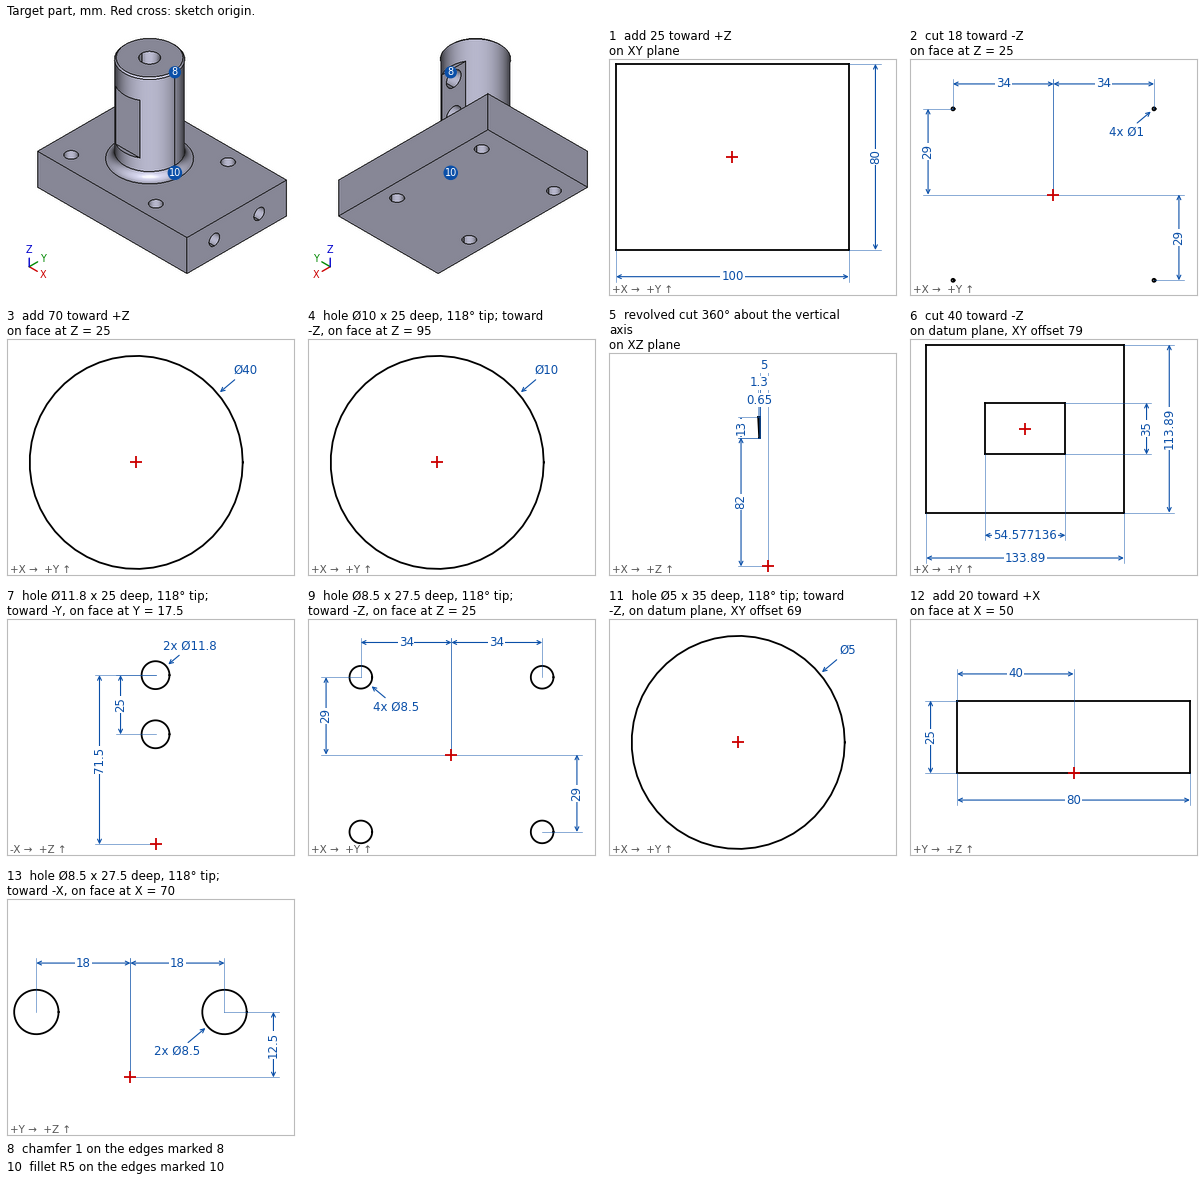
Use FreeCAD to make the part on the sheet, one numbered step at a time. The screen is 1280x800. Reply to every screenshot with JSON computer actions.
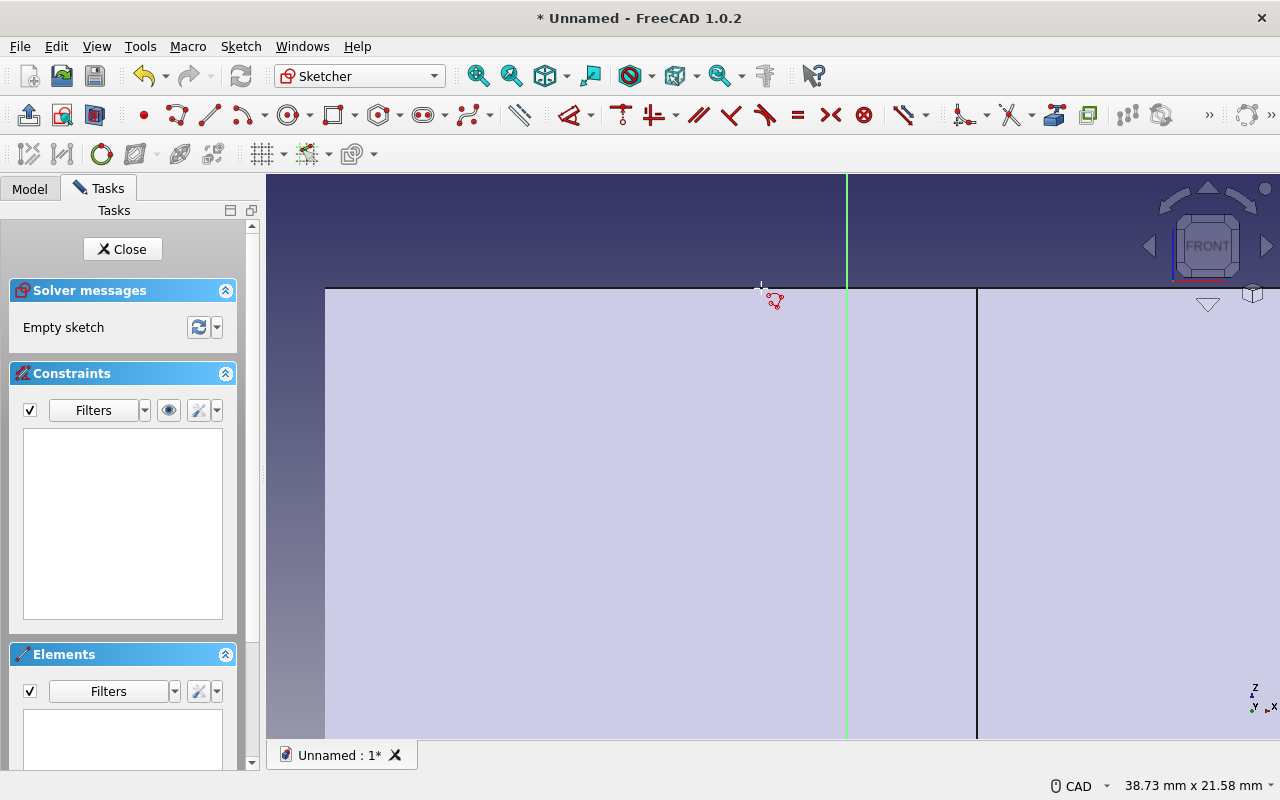
{"action": "left_click", "coordinate": [716, 628]}
{"action": "left_click", "coordinate": [699, 628]}
{"action": "left_click", "coordinate": [682, 288]}
{"action": "left_click", "coordinate": [716, 288]}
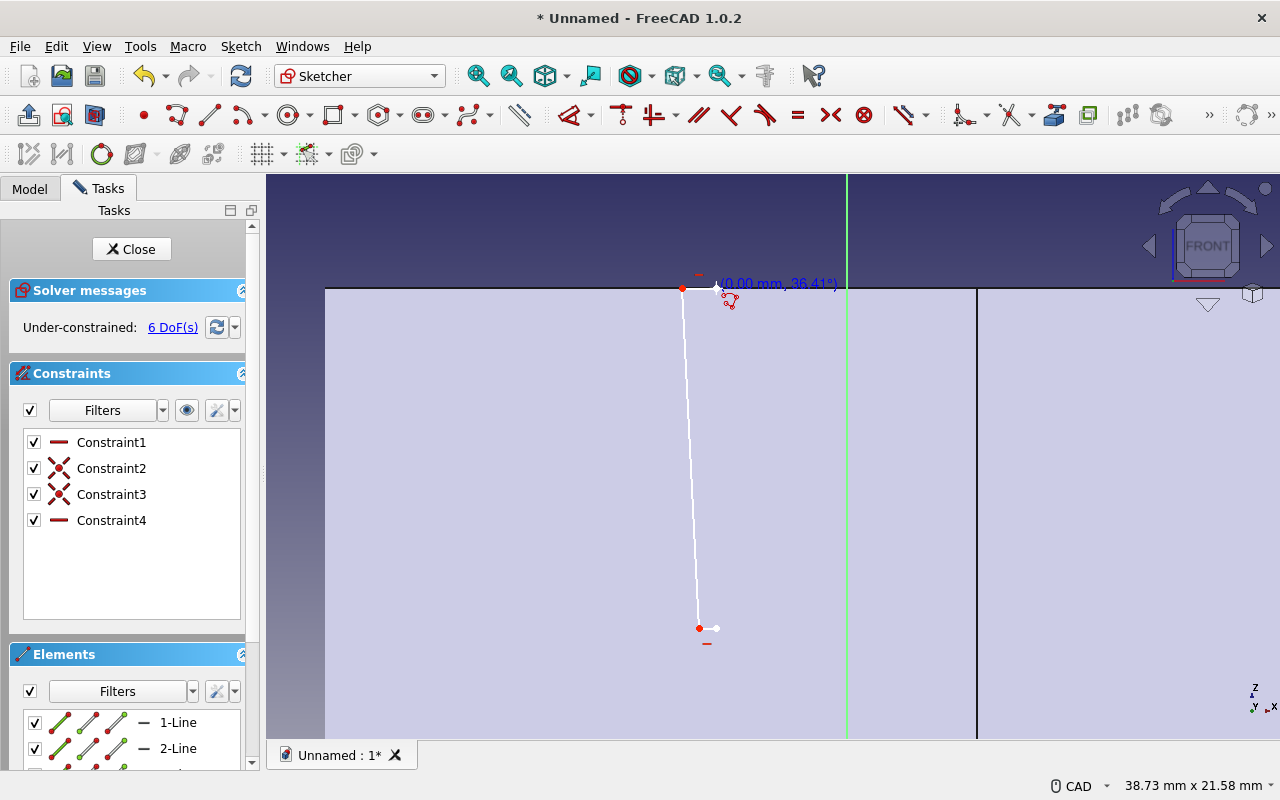
{"action": "scroll", "coordinate": [716, 628], "scroll_direction": "up", "scroll_amount": 4}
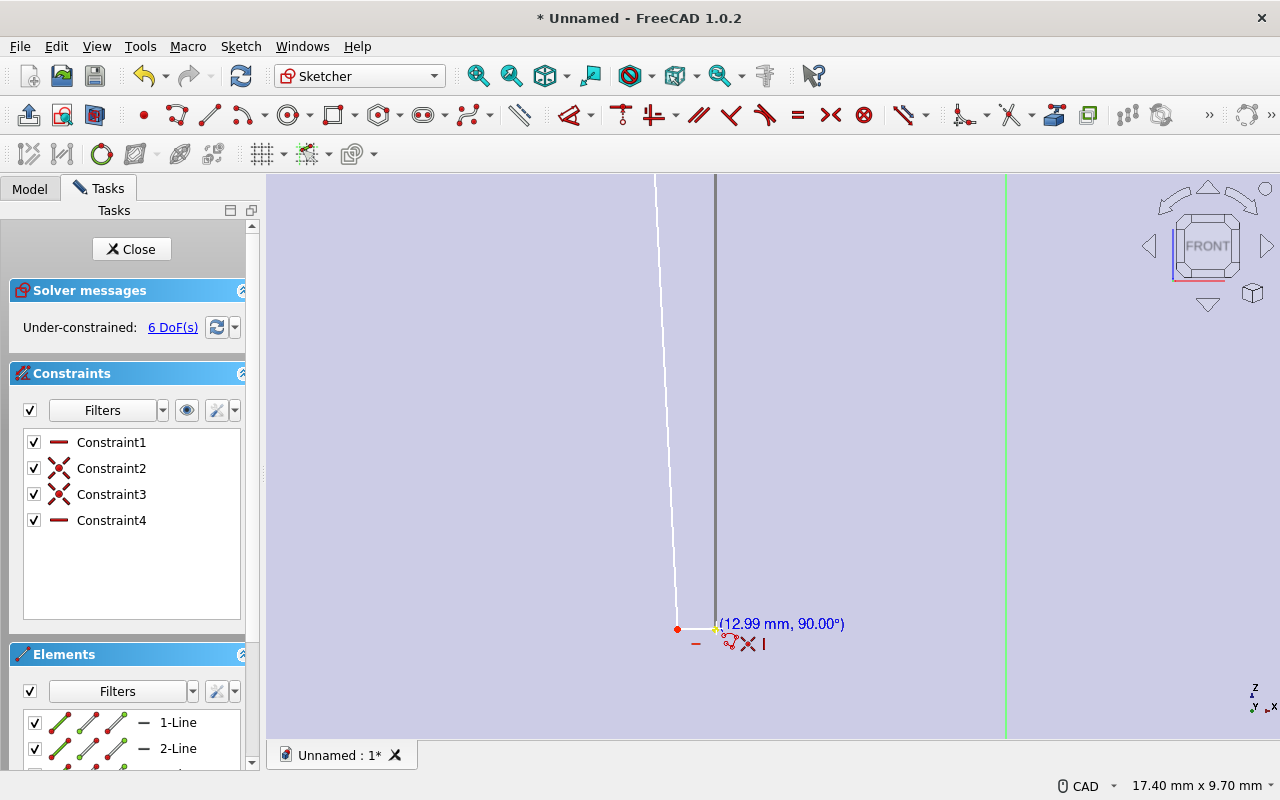
{"action": "left_click", "coordinate": [715, 629]}
{"action": "key", "text": "Escape"}
{"action": "key", "text": "Escape"}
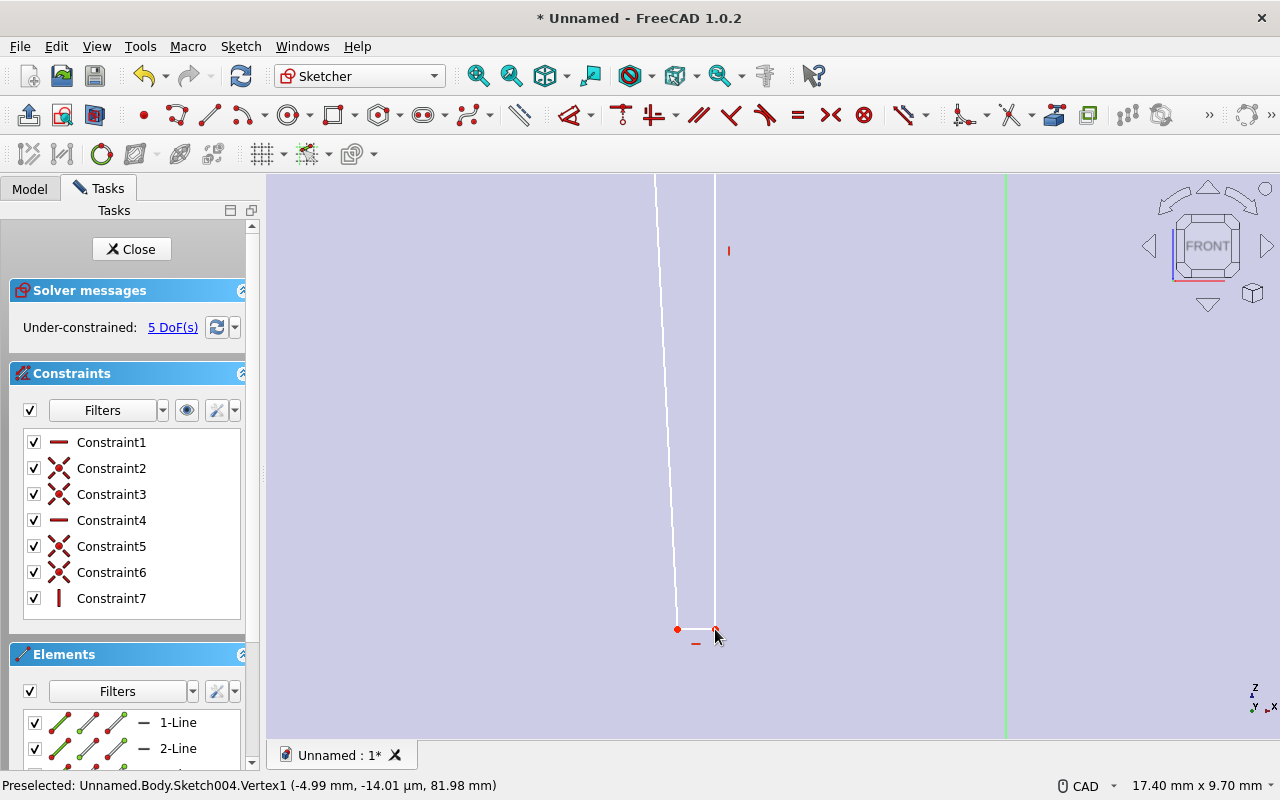
{"action": "left_click", "coordinate": [715, 402]}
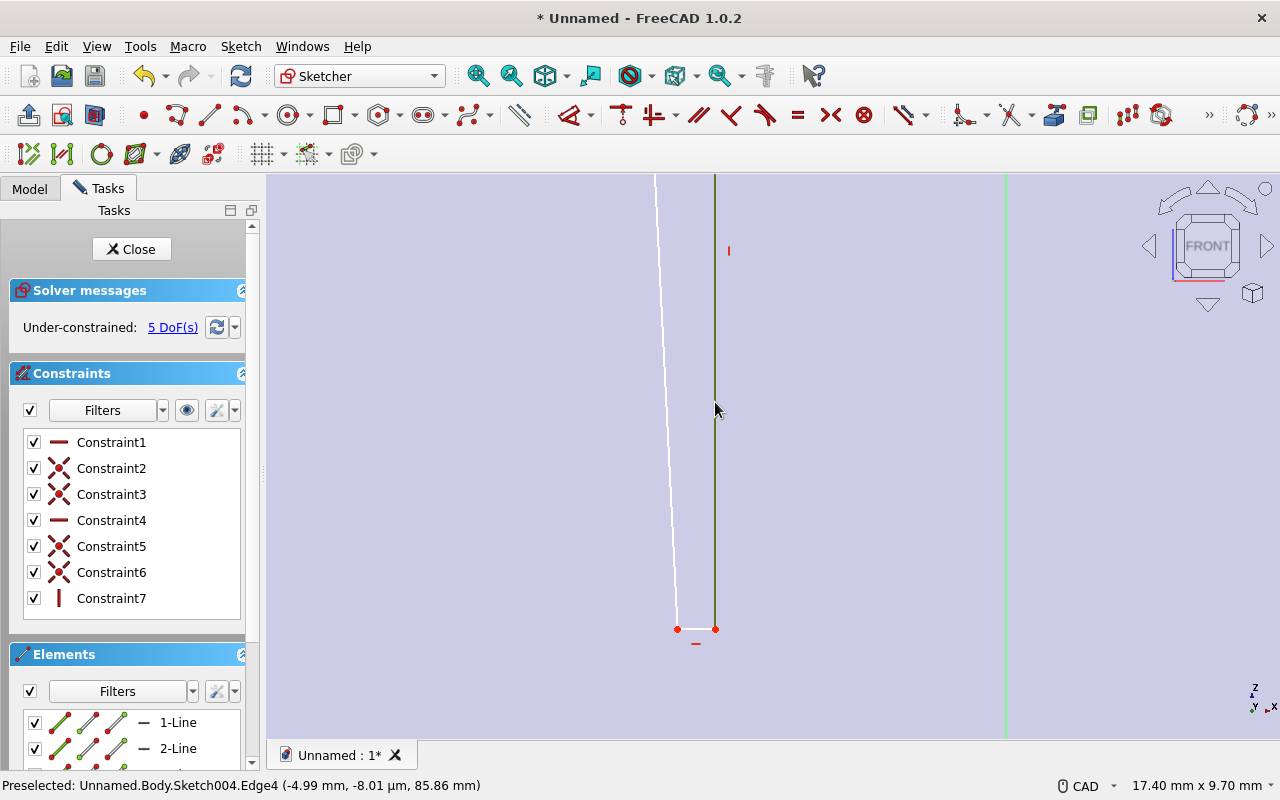
{"action": "key", "text": "i"}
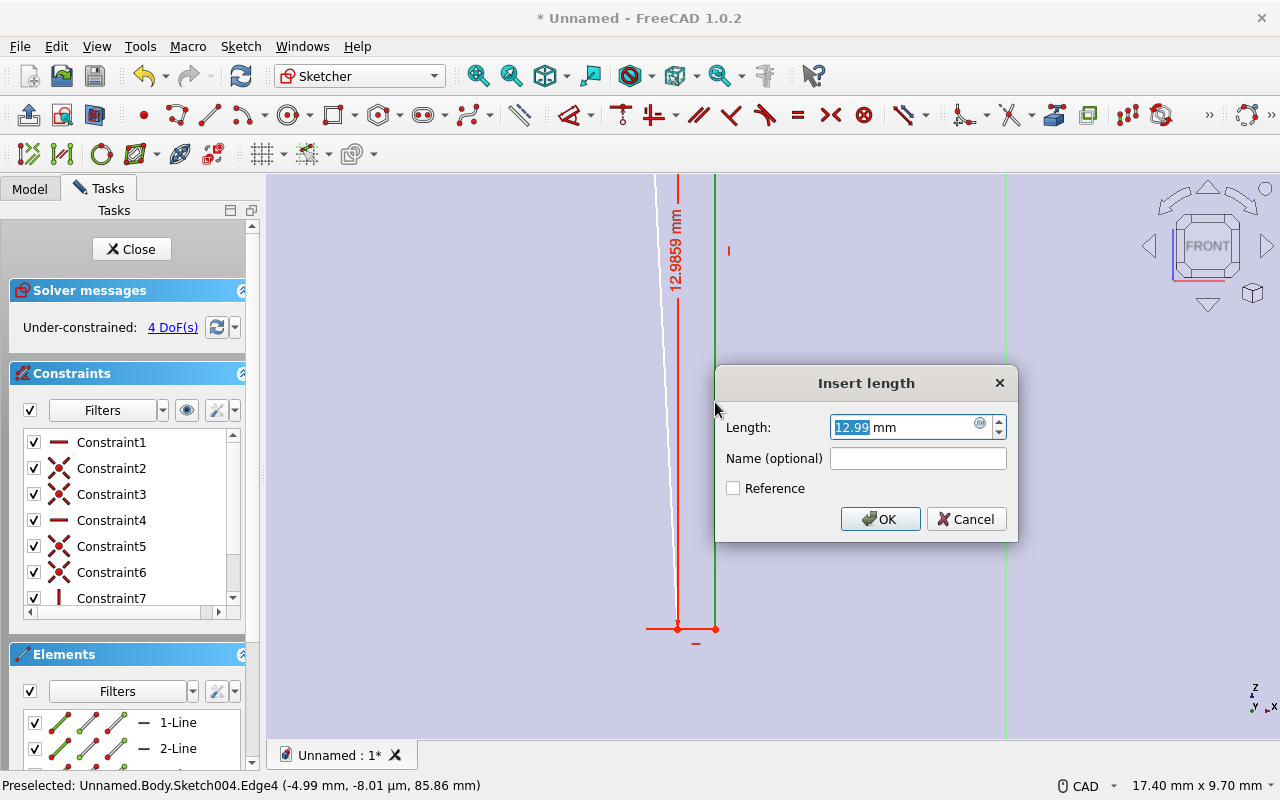
{"action": "type", "text": "13"}
{"action": "key", "text": "Return"}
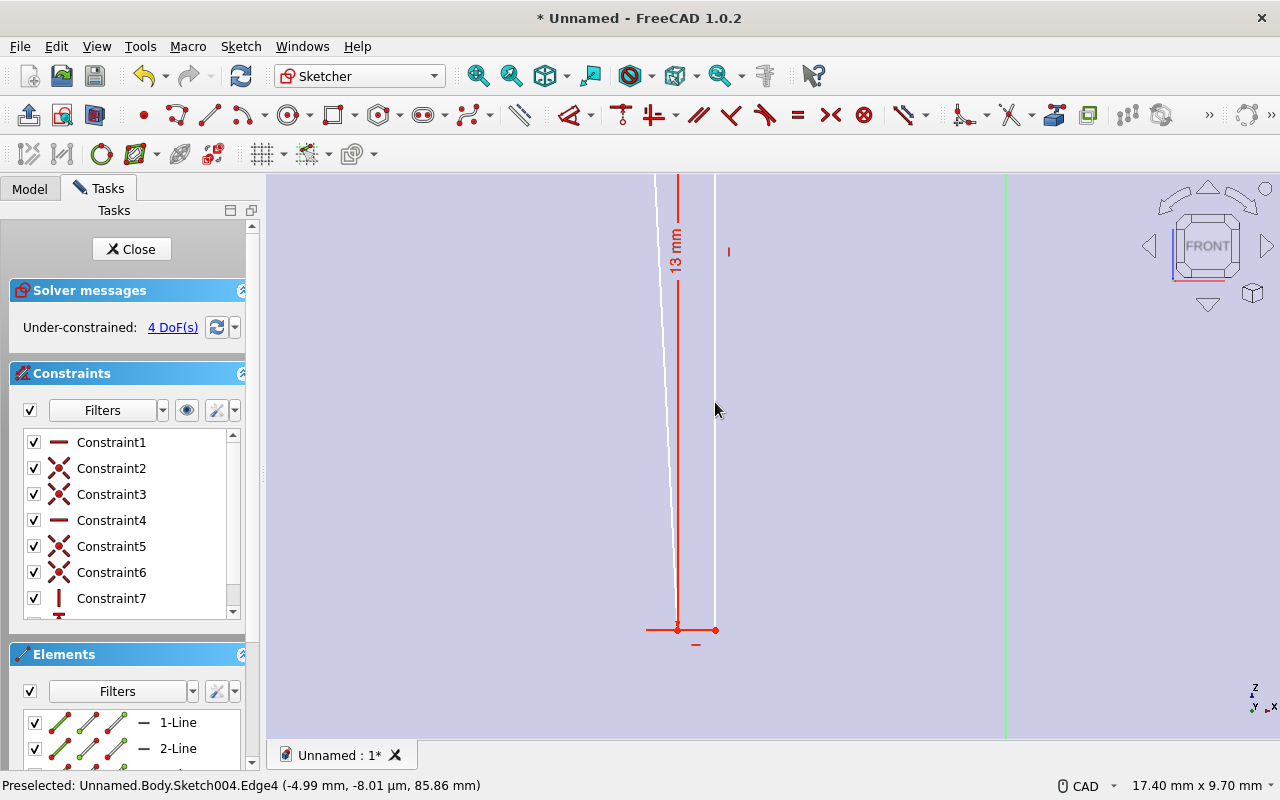
{"action": "left_click", "coordinate": [715, 630]}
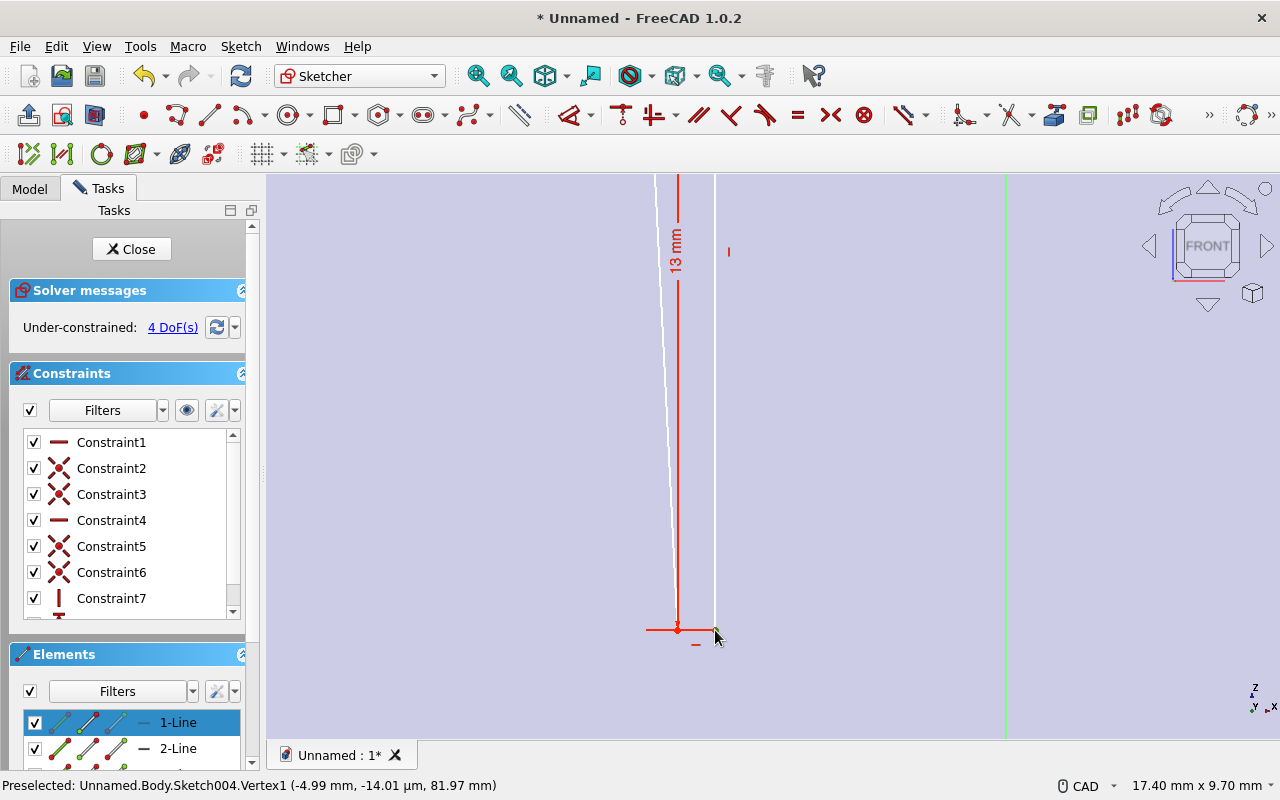
{"action": "left_click", "coordinate": [590, 116]}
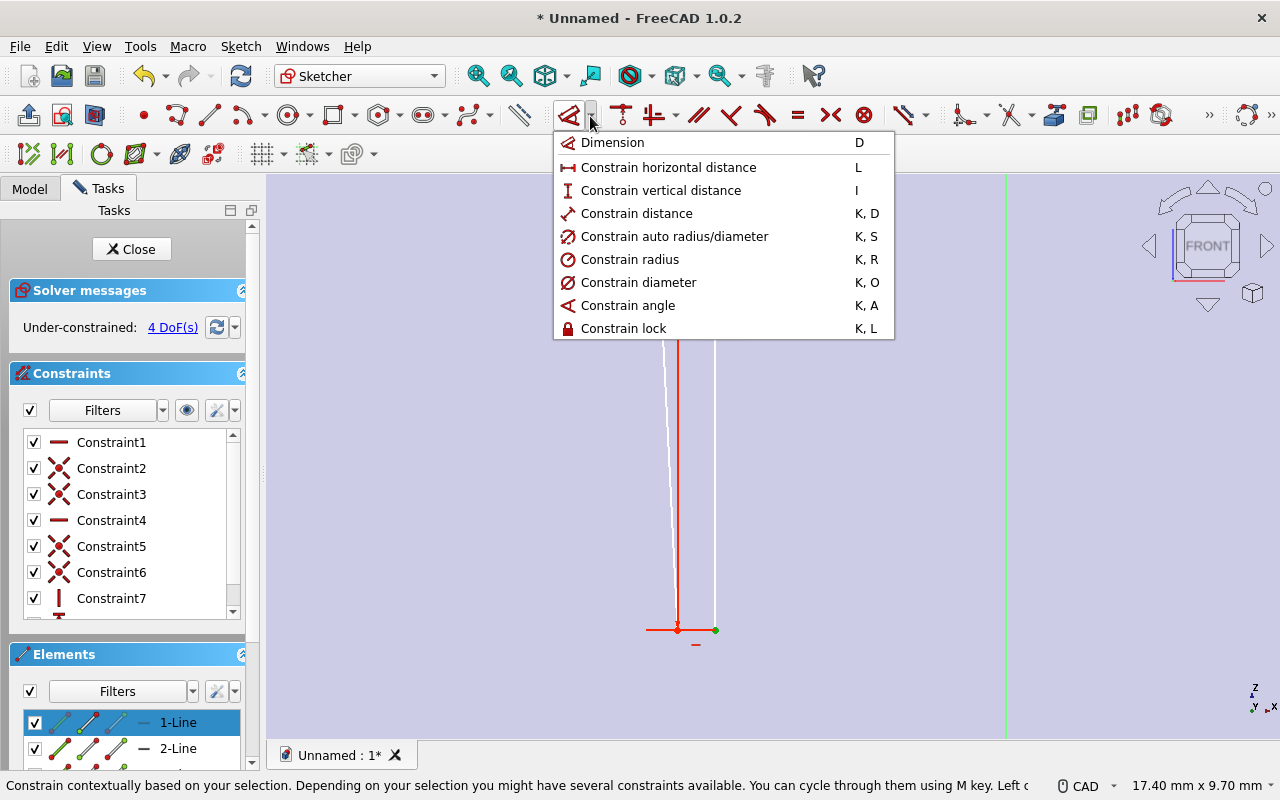
{"action": "left_click", "coordinate": [724, 168]}